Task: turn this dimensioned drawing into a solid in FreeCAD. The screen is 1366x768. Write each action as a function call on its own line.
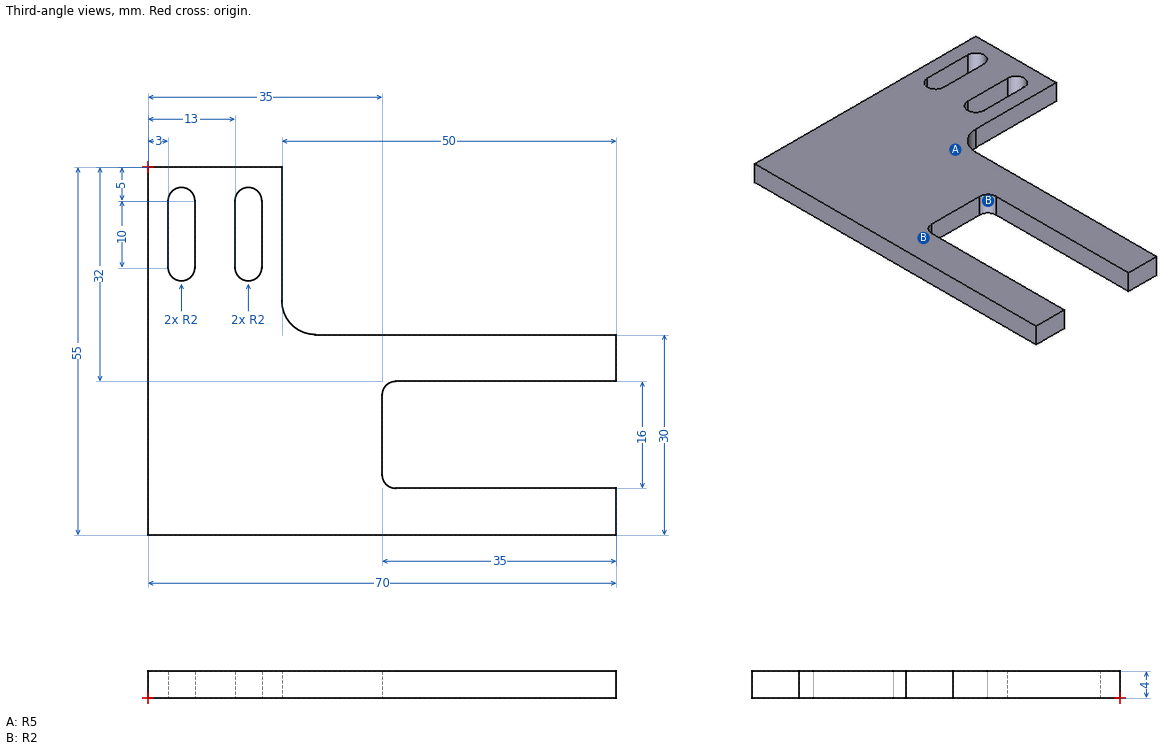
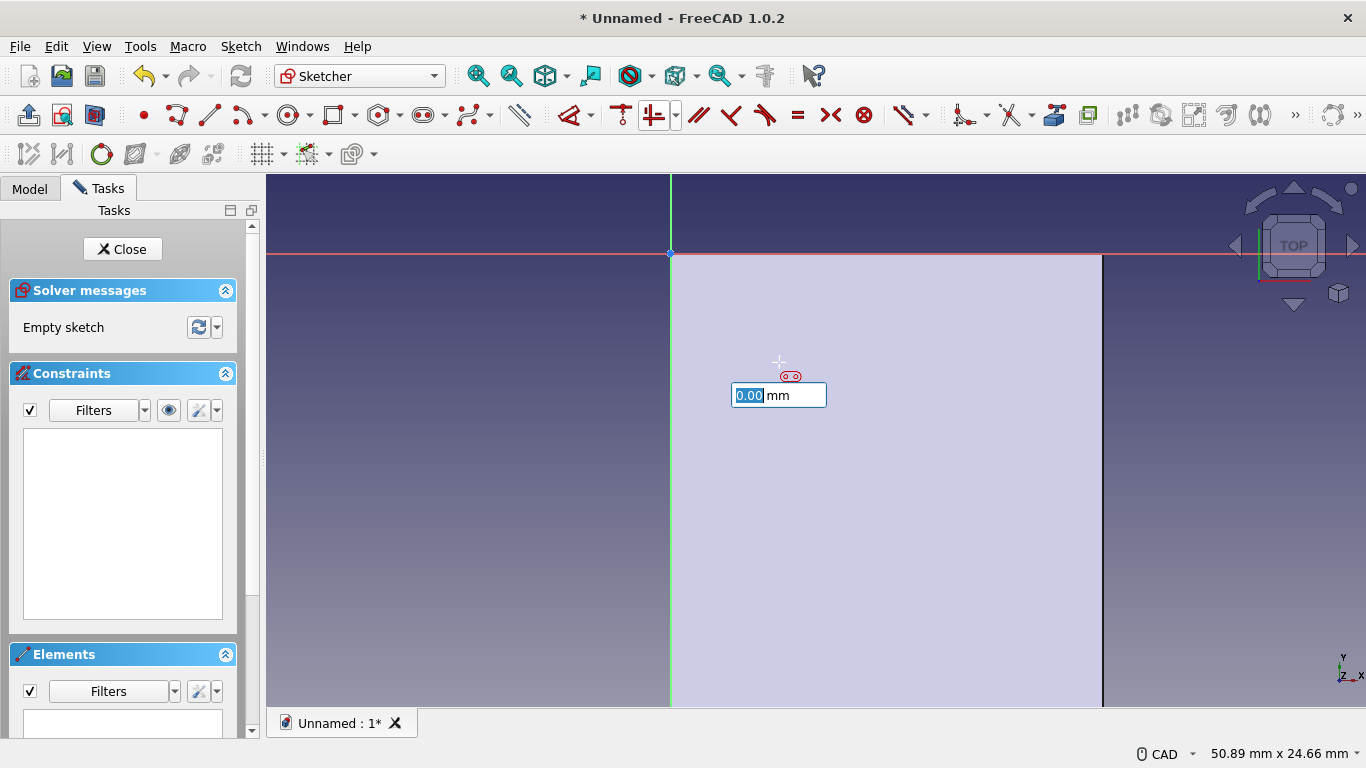
click(736, 470)
key(Escape)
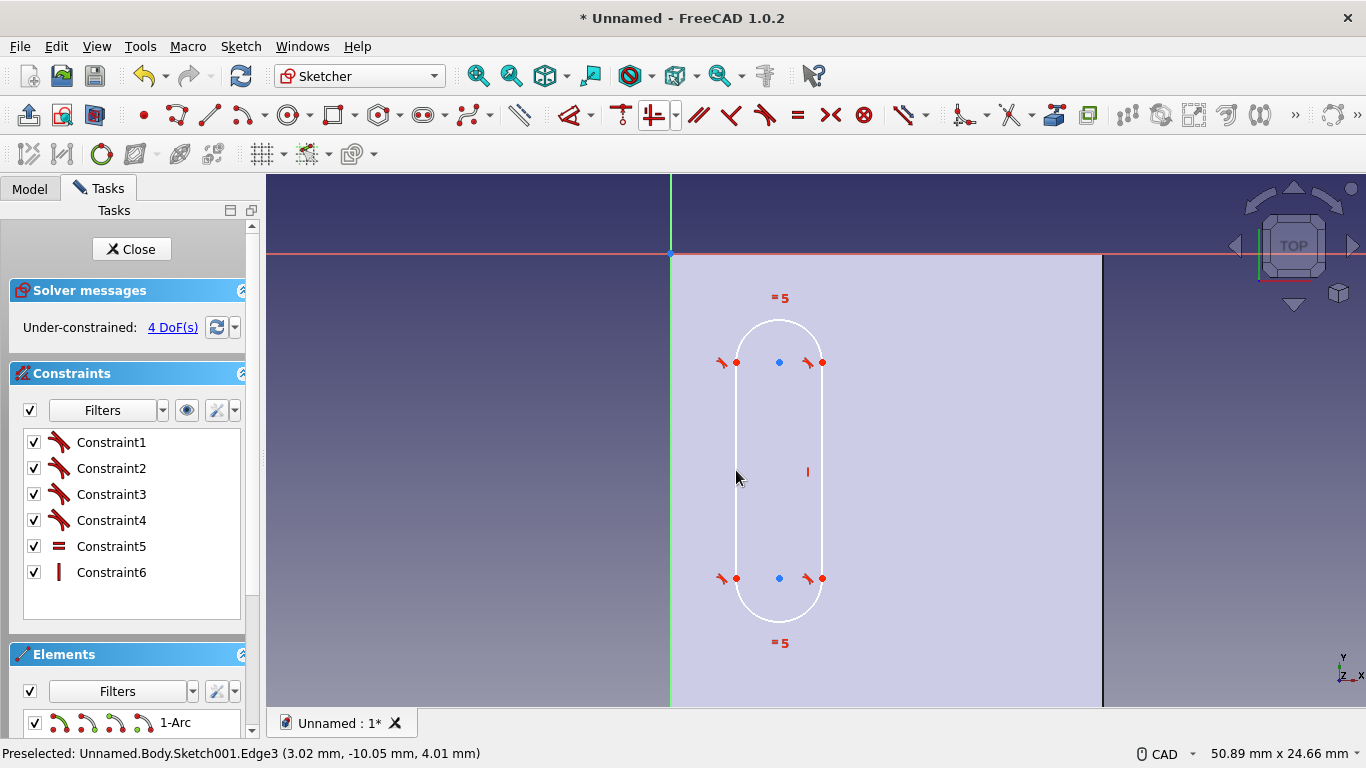
click(568, 116)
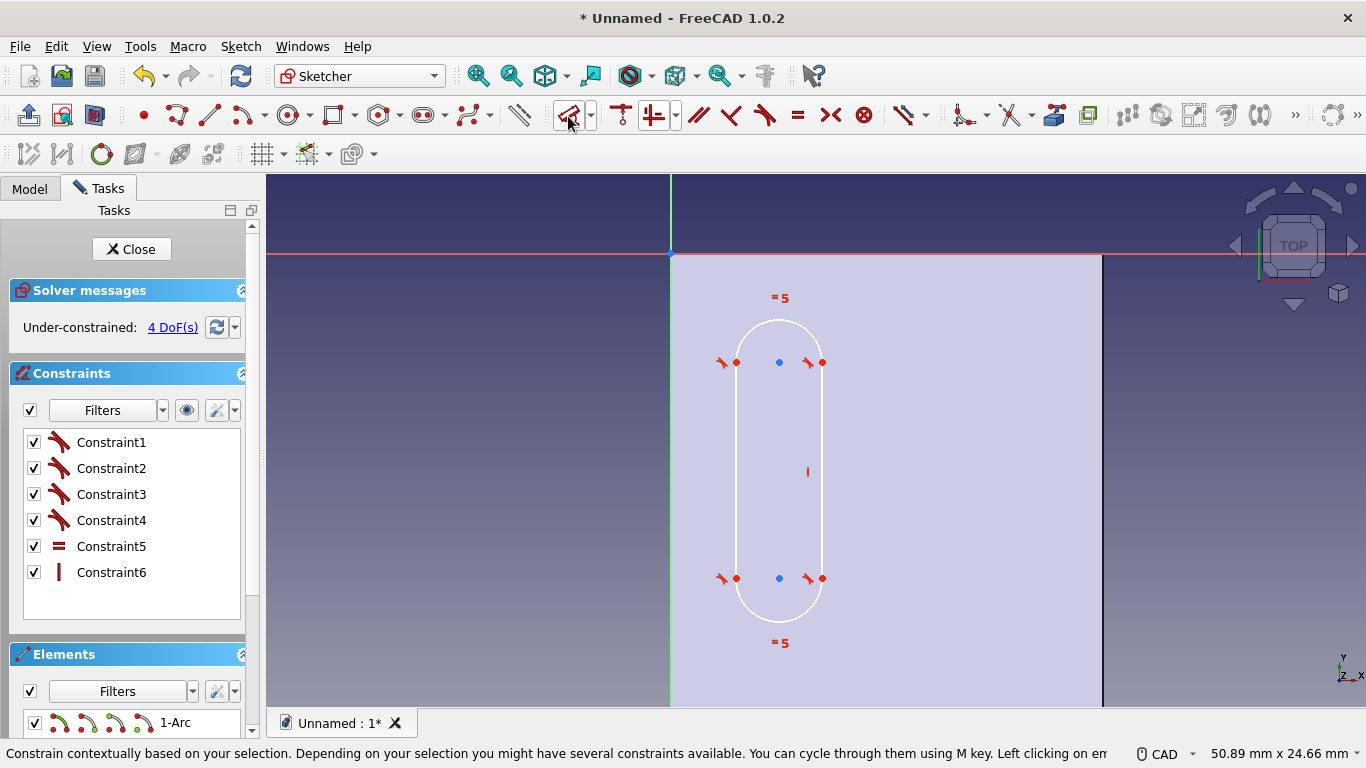
click(754, 614)
click(735, 640)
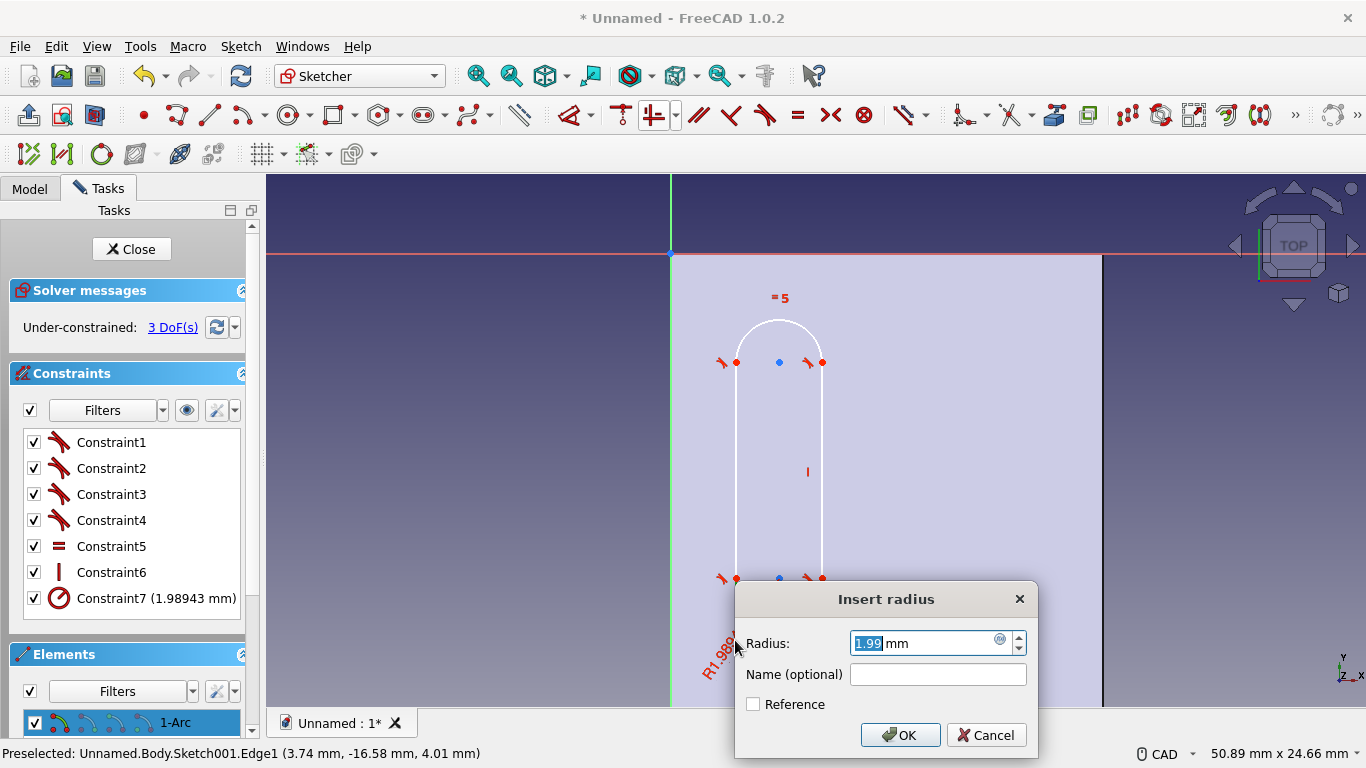
text(2)
key(Return)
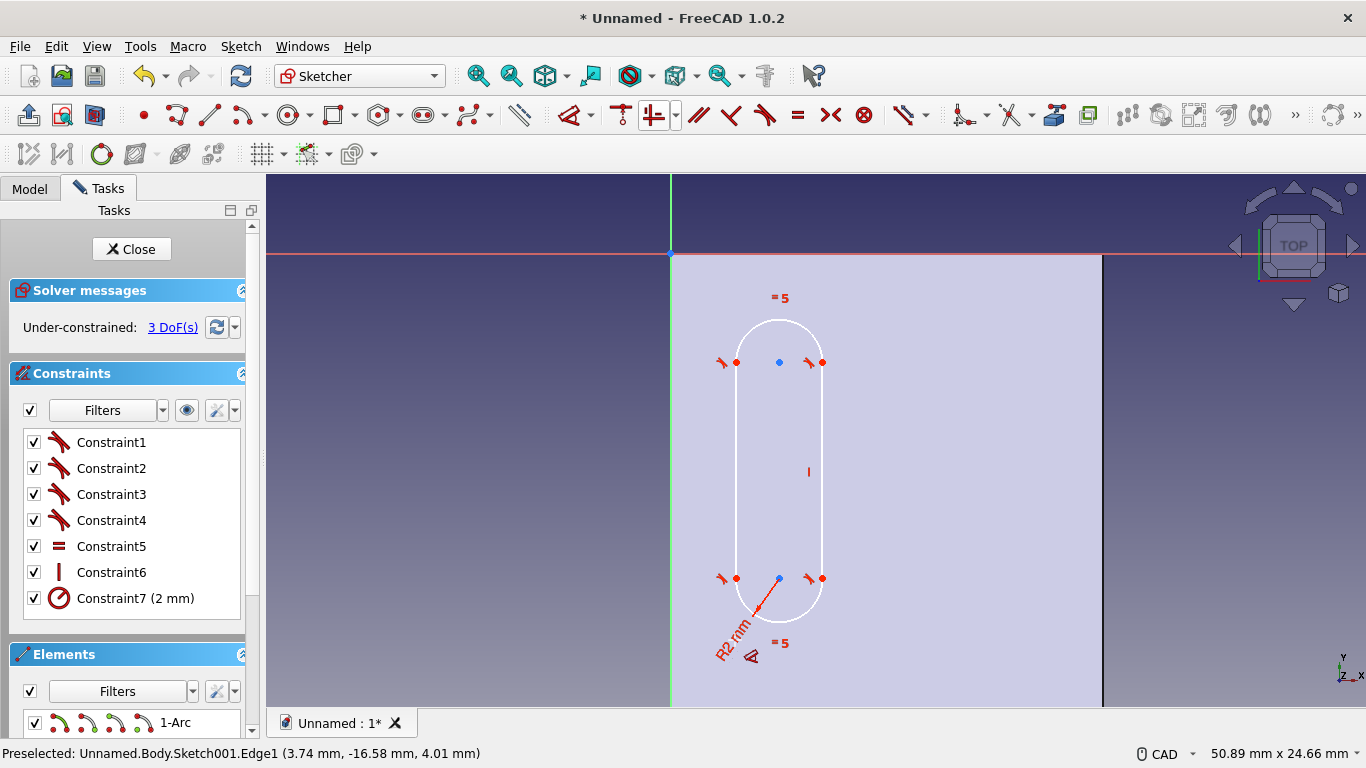
click(736, 514)
click(702, 471)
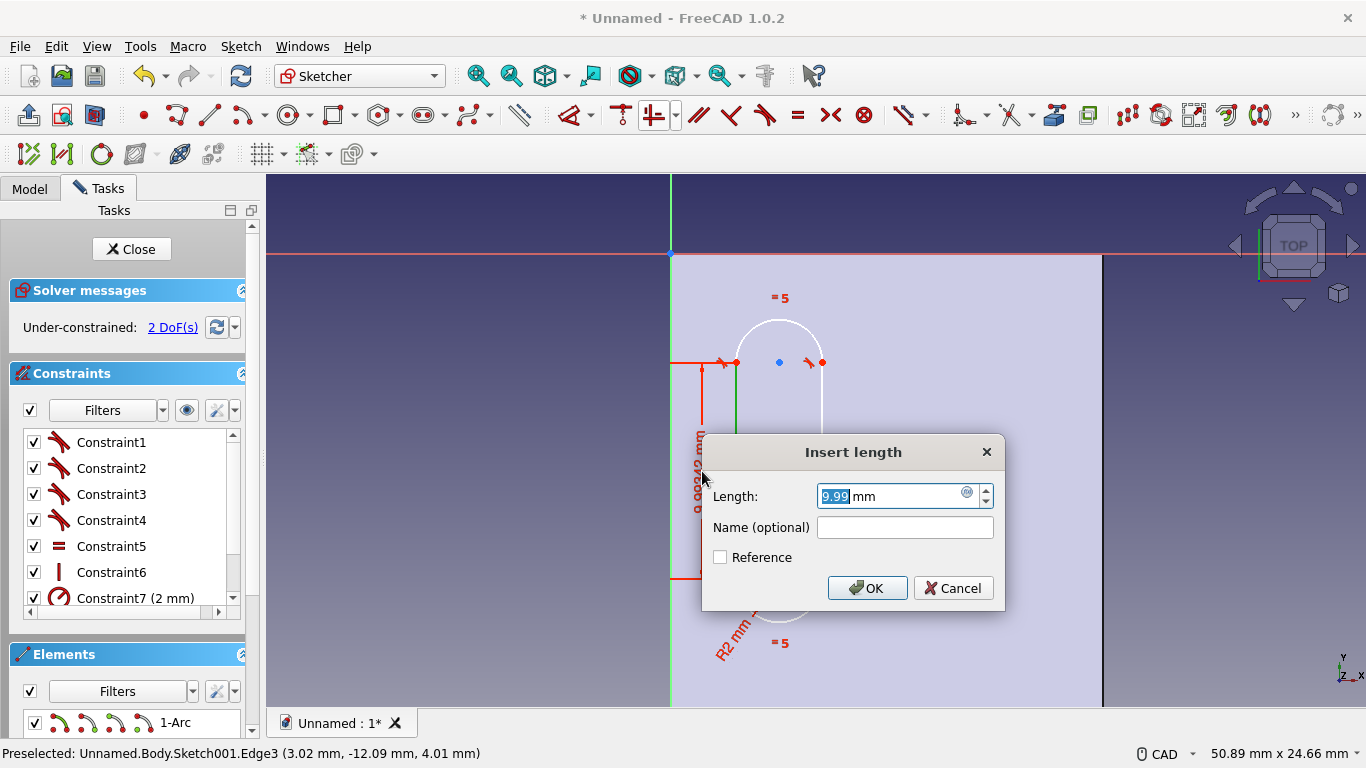
text(10)
key(Return)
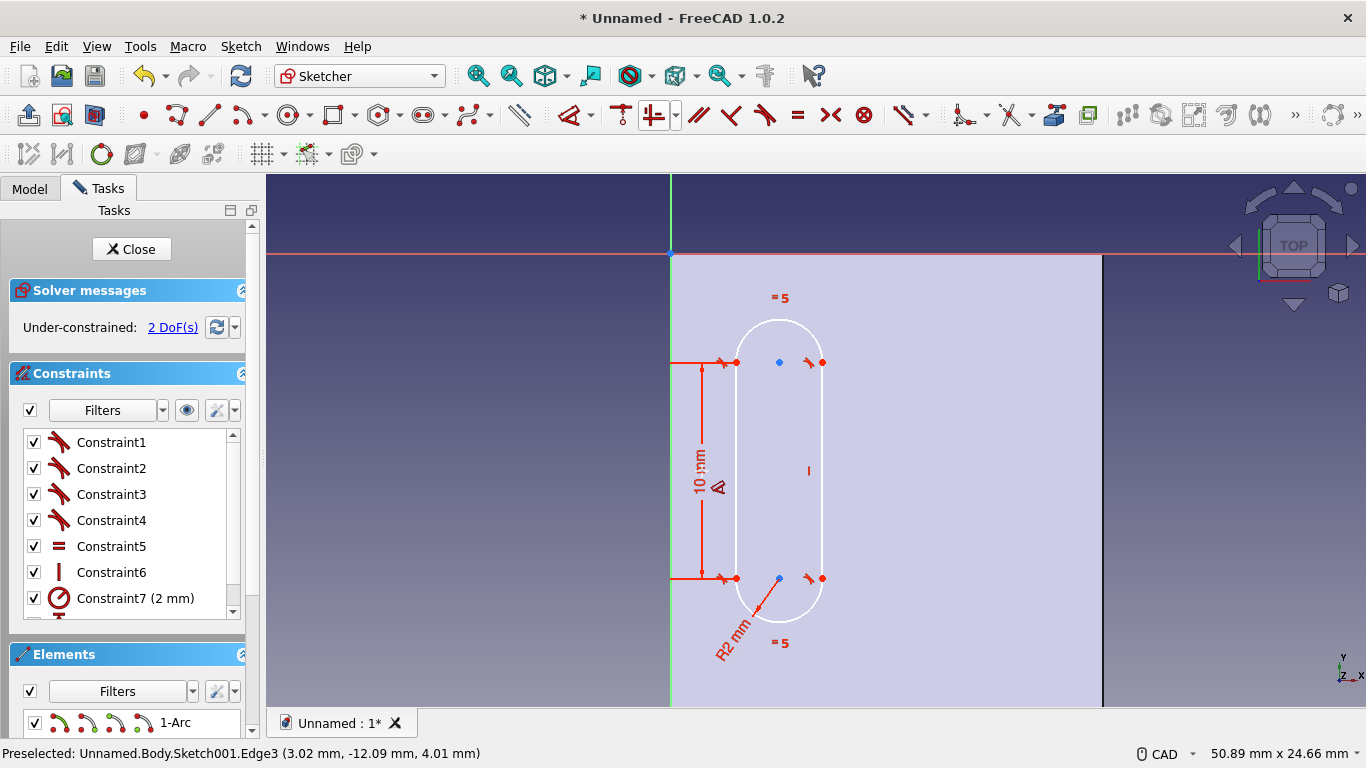
click(736, 579)
click(703, 220)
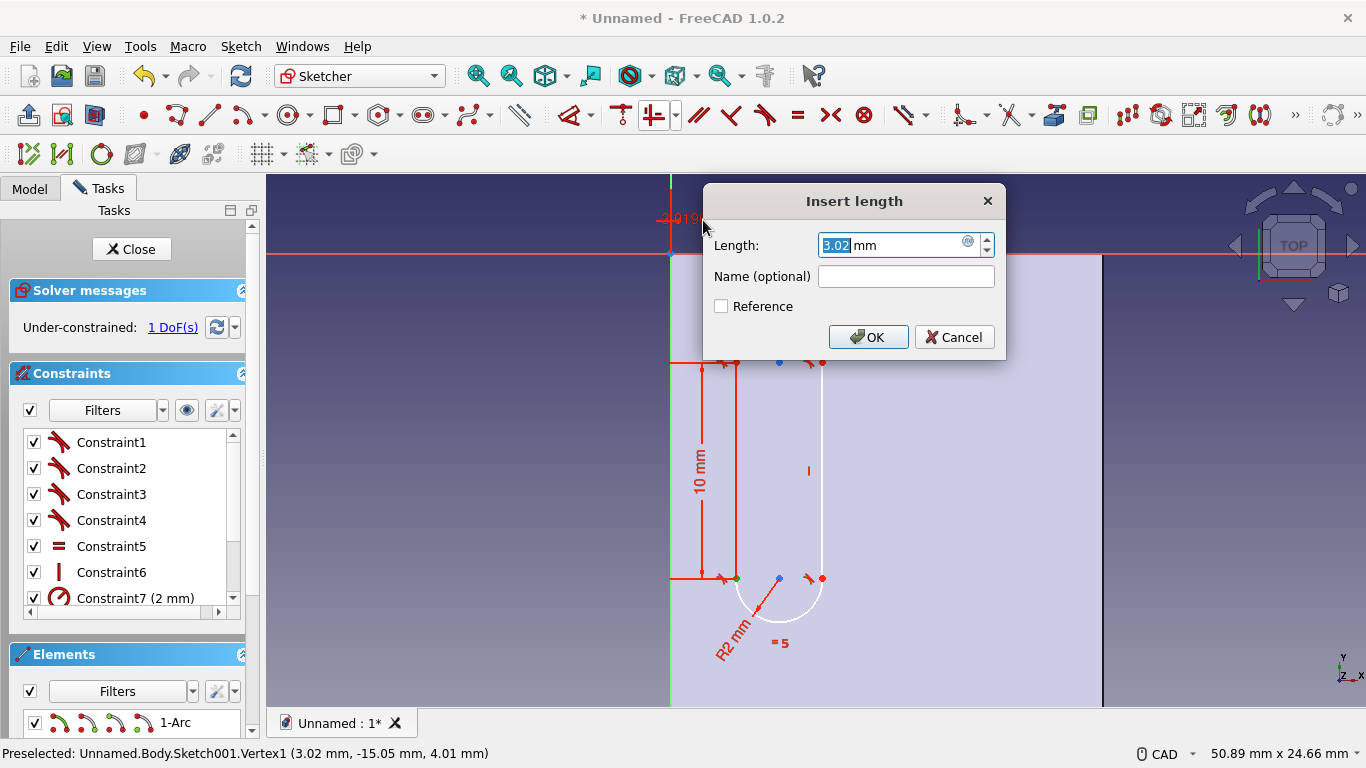
text(3)
key(Return)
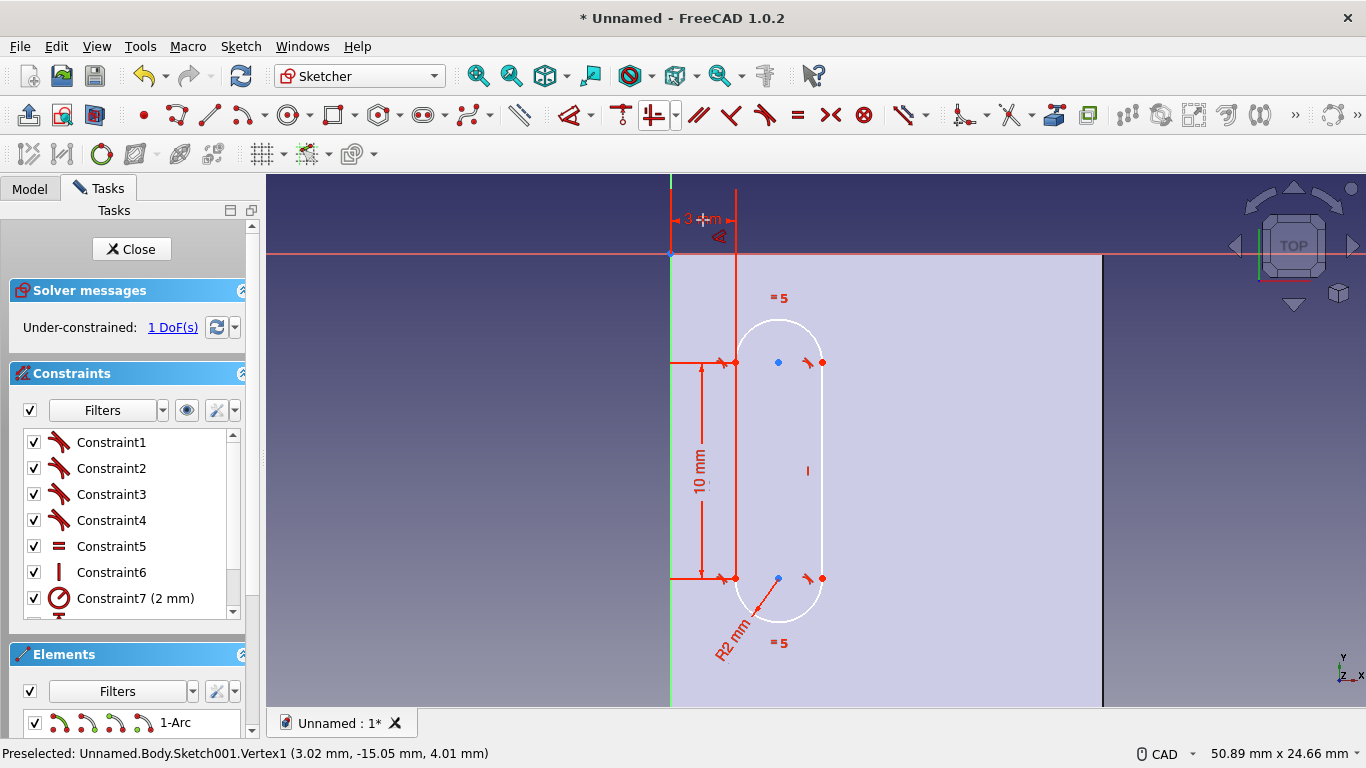
click(822, 363)
click(856, 308)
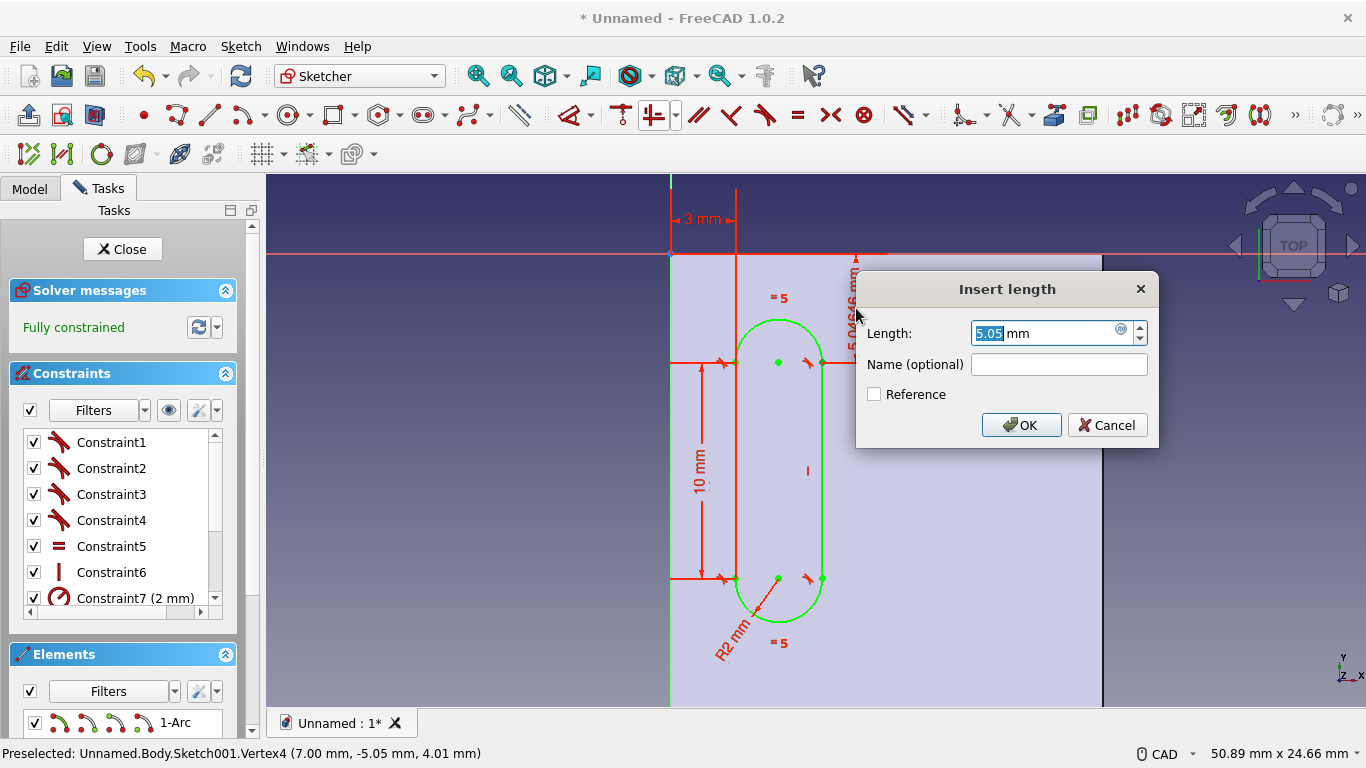
text(5)
key(Return)
key(Escape)